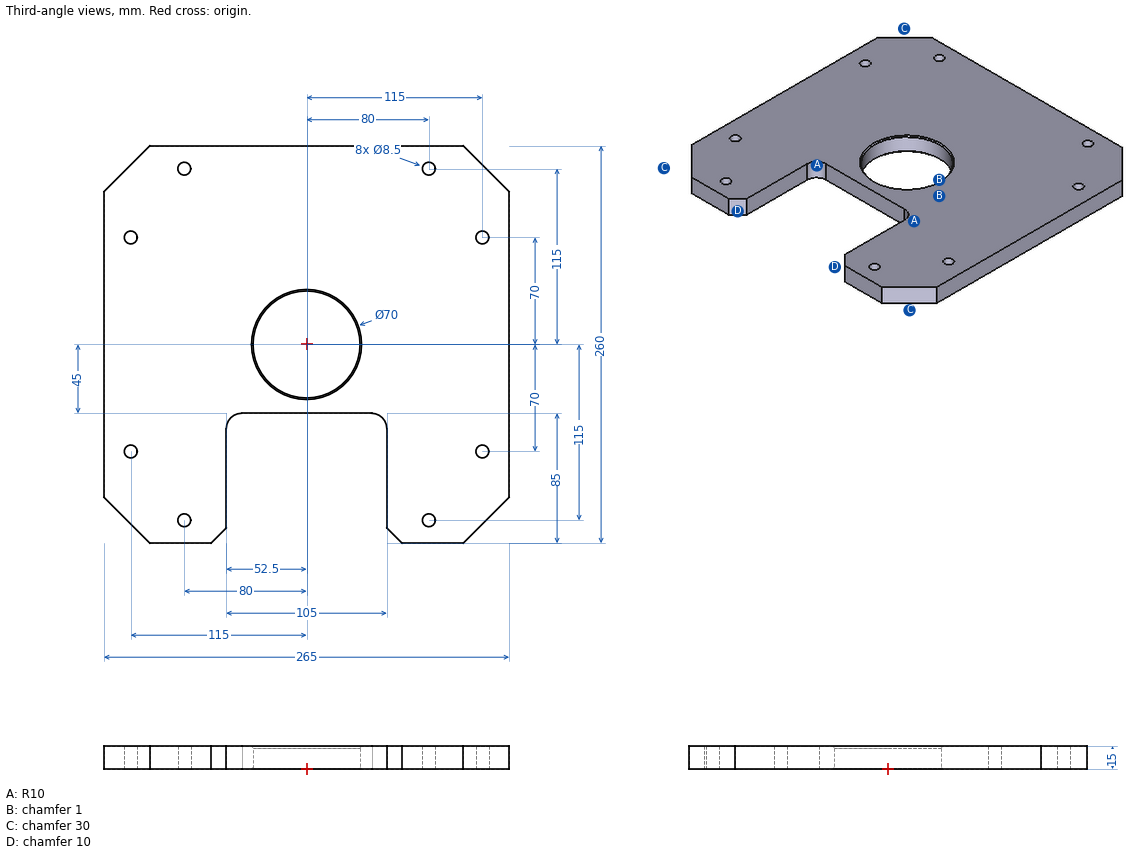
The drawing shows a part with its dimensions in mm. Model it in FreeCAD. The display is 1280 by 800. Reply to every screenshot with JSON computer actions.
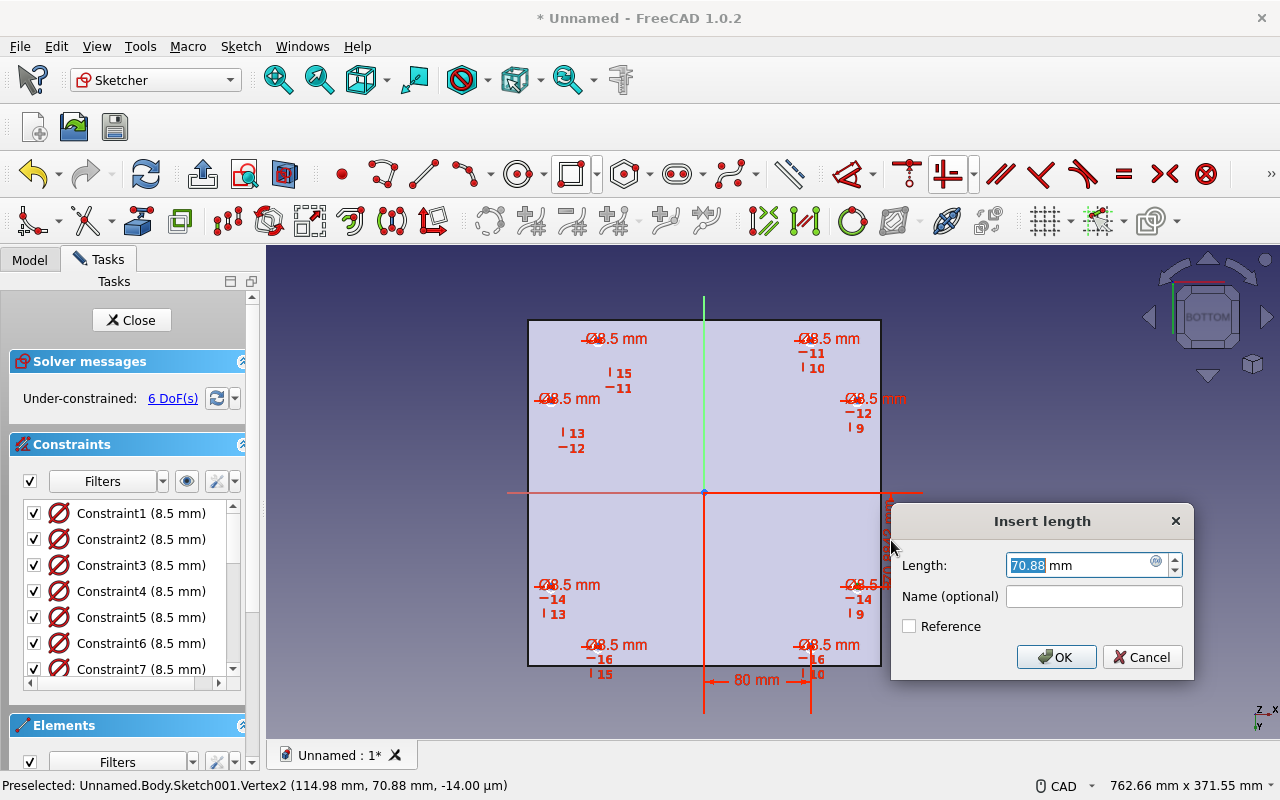
{"action": "type", "text": "70"}
{"action": "key", "text": "Return"}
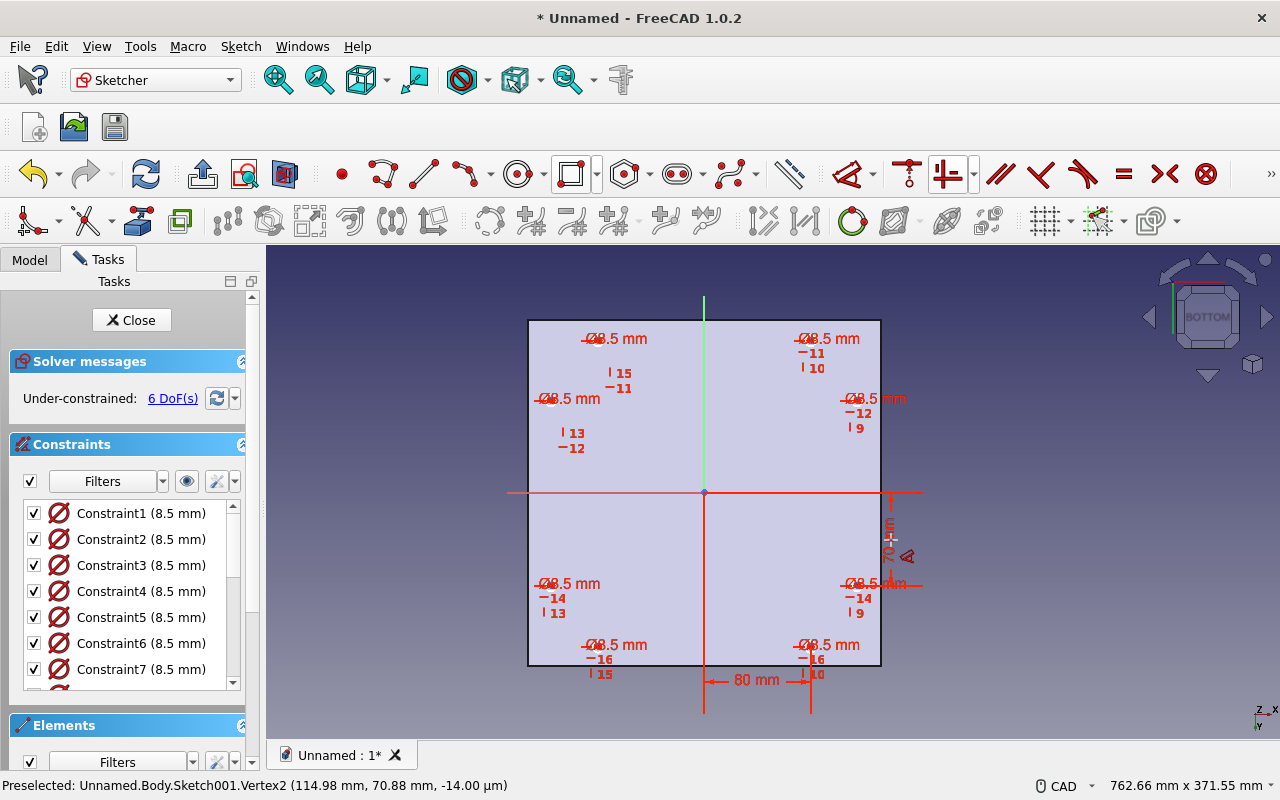
{"action": "left_click", "coordinate": [857, 401]}
{"action": "left_click", "coordinate": [891, 447]}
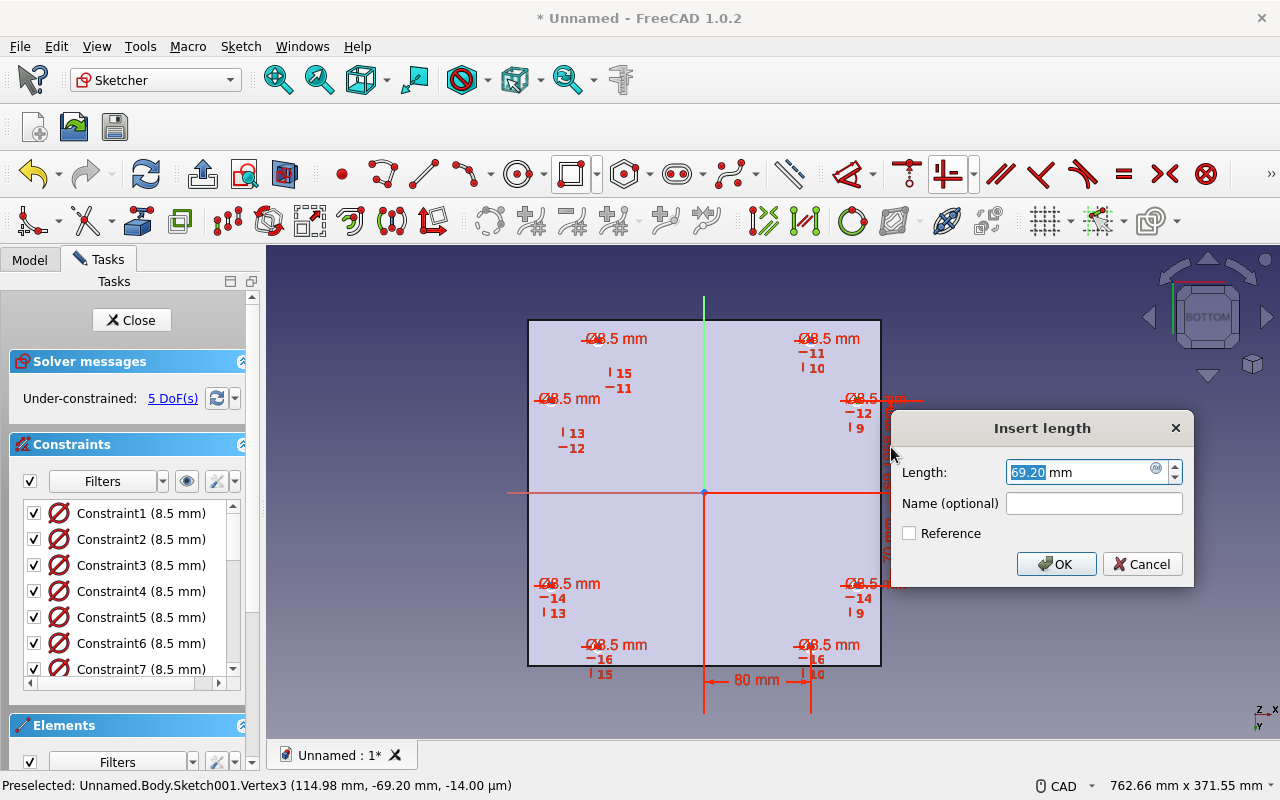
{"action": "type", "text": "70"}
{"action": "key", "text": "Return"}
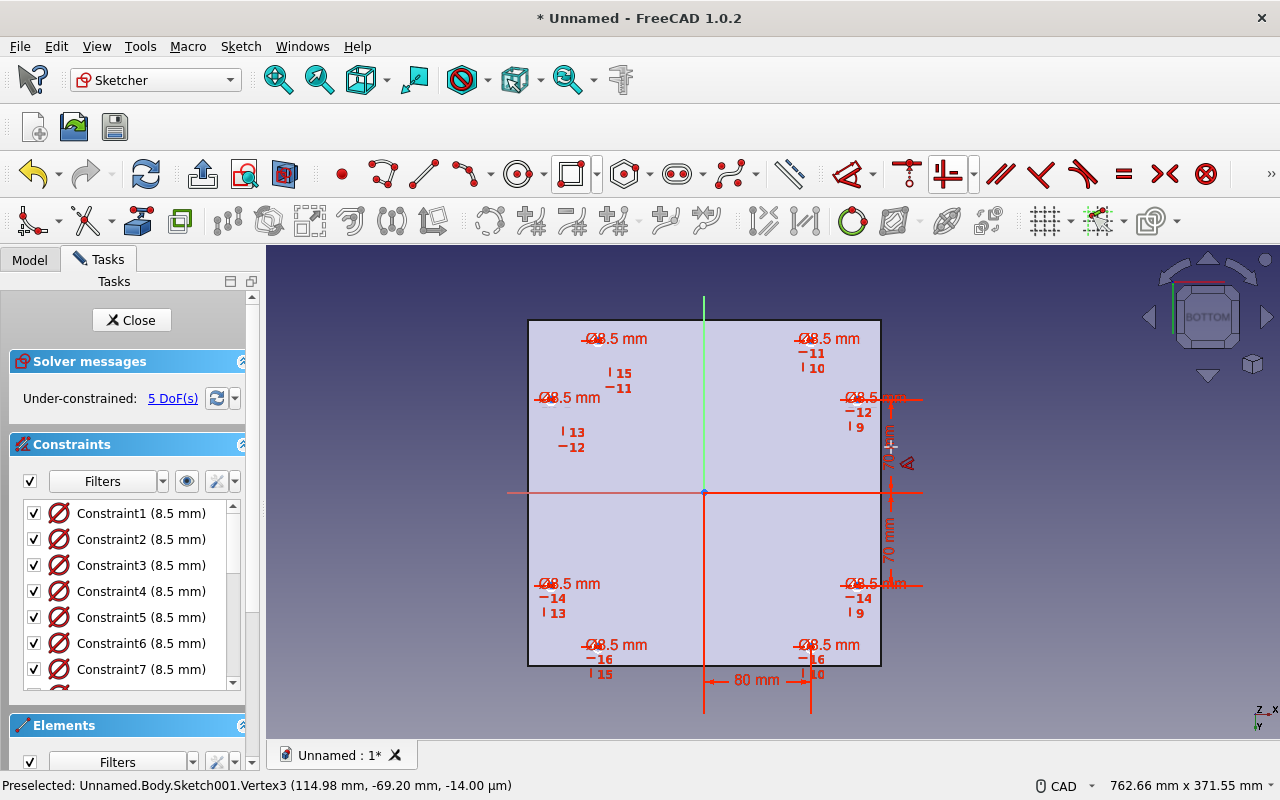
{"action": "left_click", "coordinate": [598, 341]}
{"action": "left_click", "coordinate": [651, 307]}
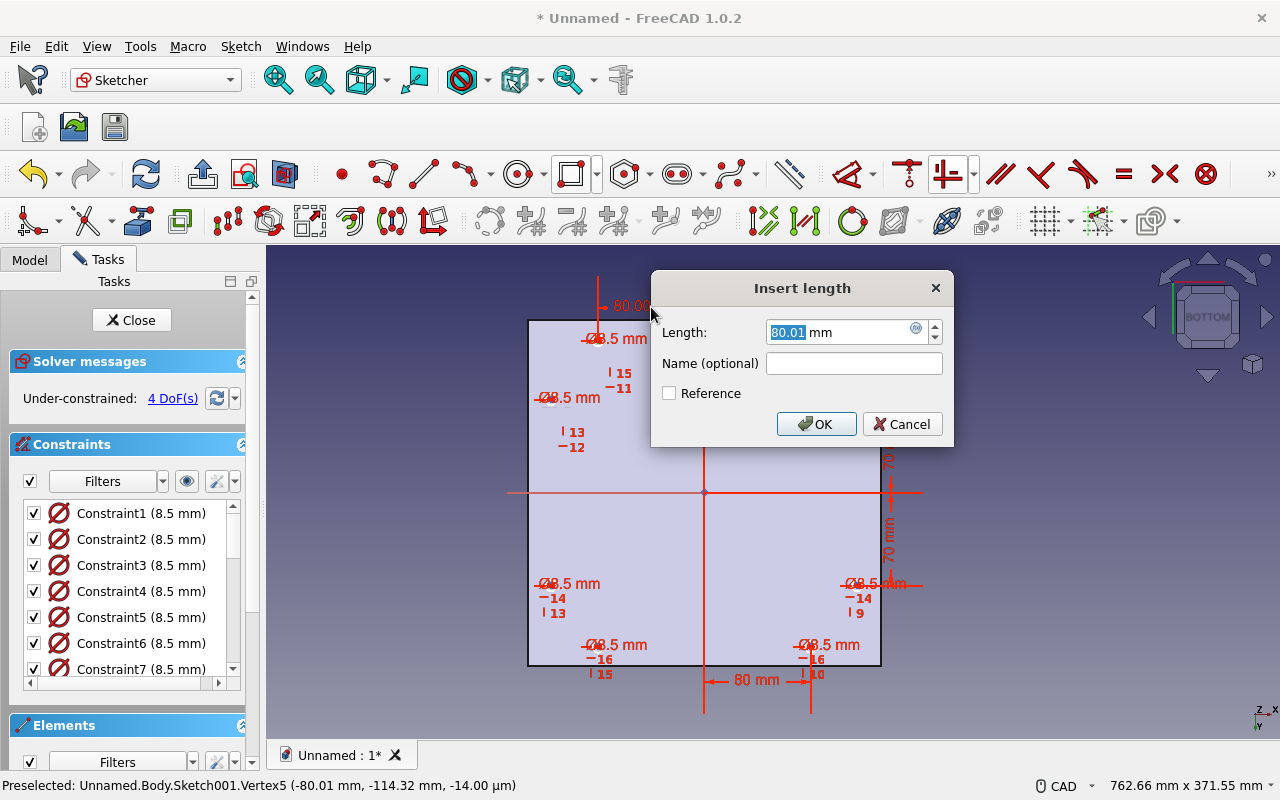
{"action": "type", "text": "80"}
{"action": "key", "text": "Return"}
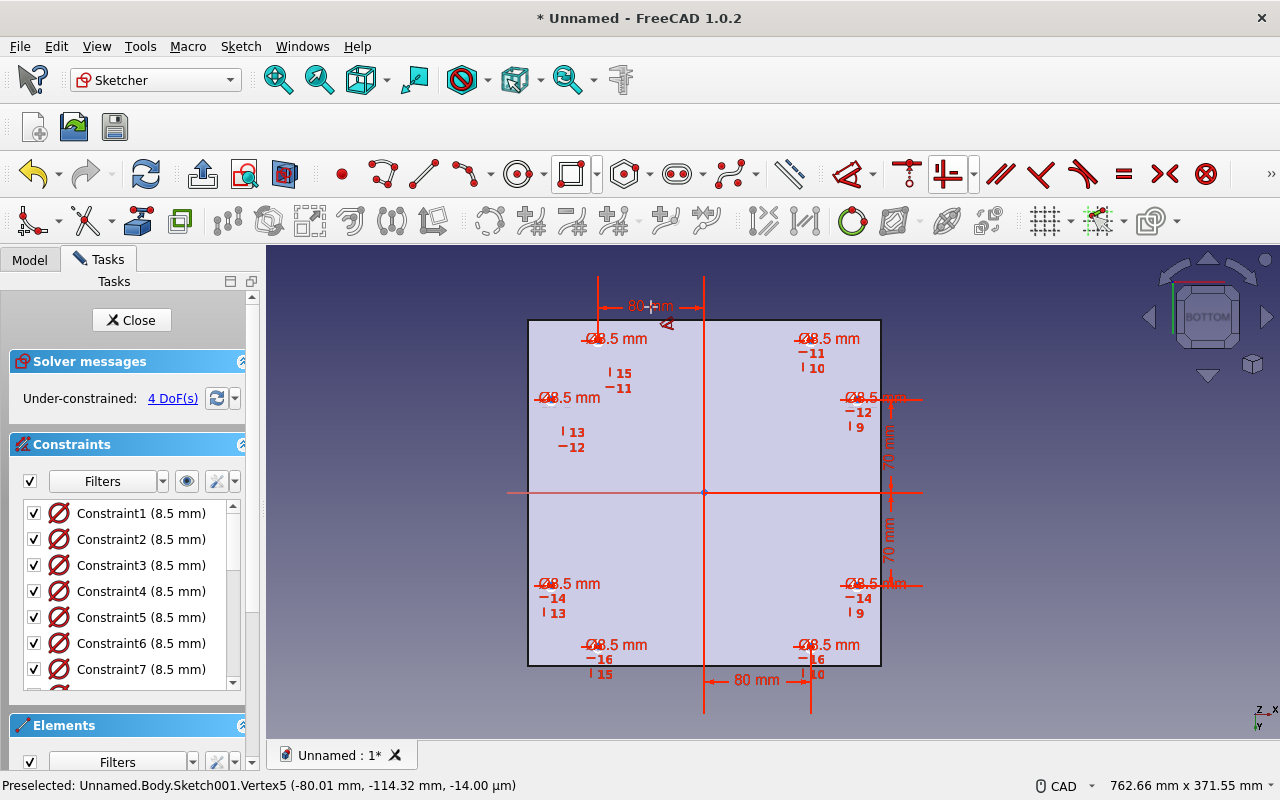
{"action": "left_click", "coordinate": [811, 647]}
{"action": "left_click", "coordinate": [845, 570]}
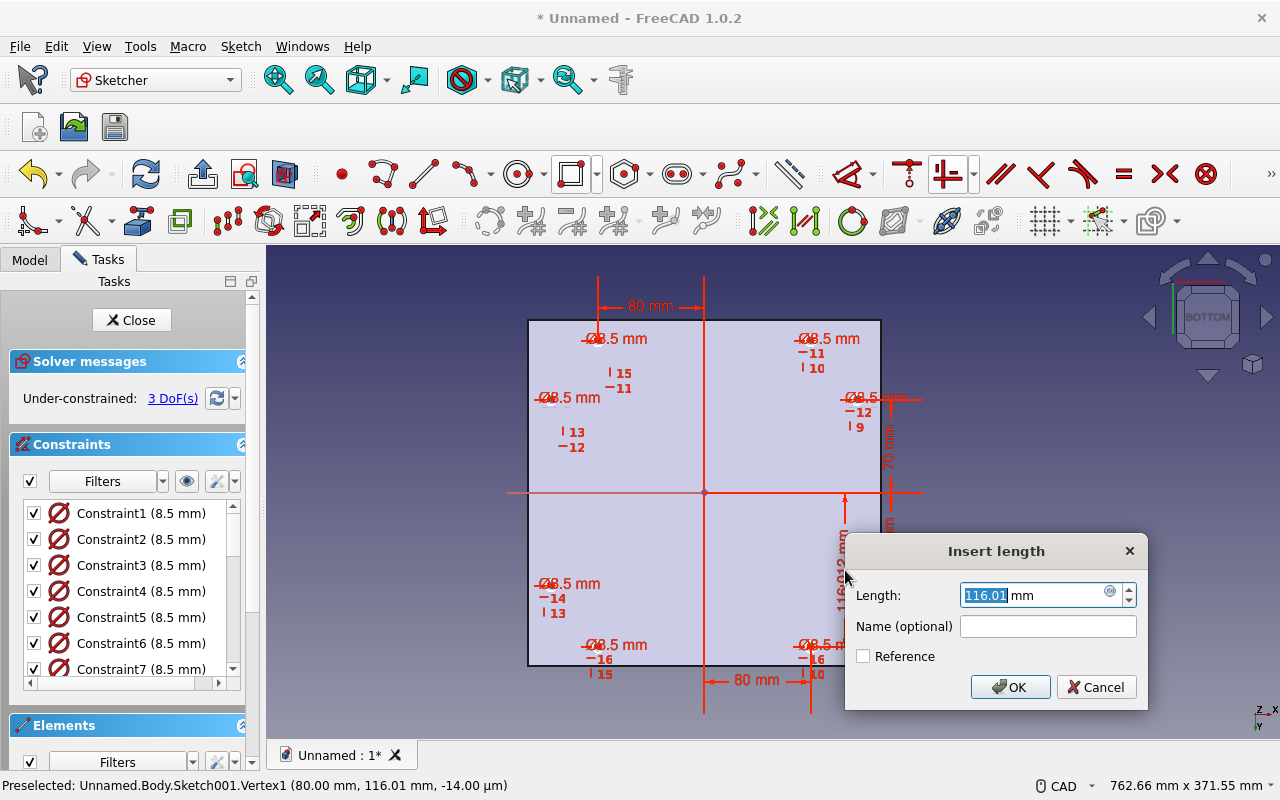
{"action": "type", "text": "115"}
{"action": "key", "text": "Return"}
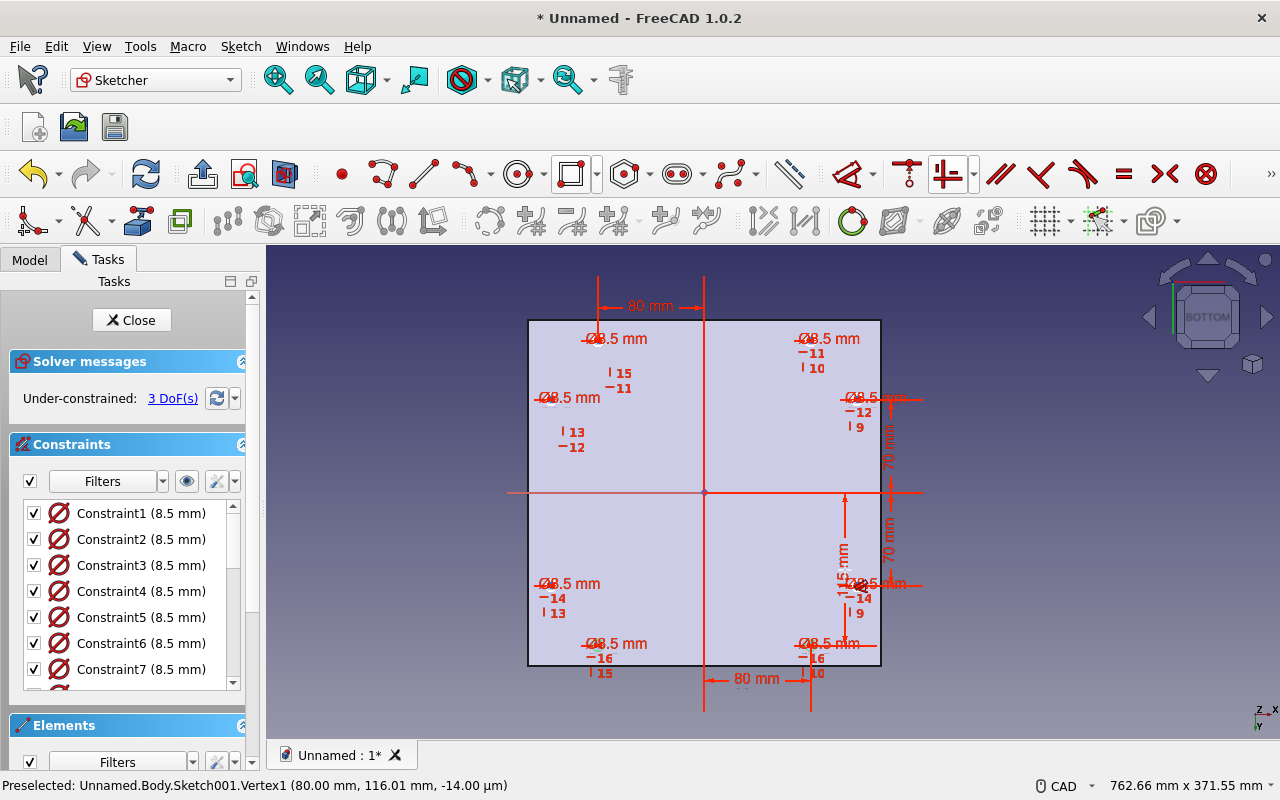
{"action": "left_click", "coordinate": [857, 586]}
{"action": "left_click", "coordinate": [781, 620]}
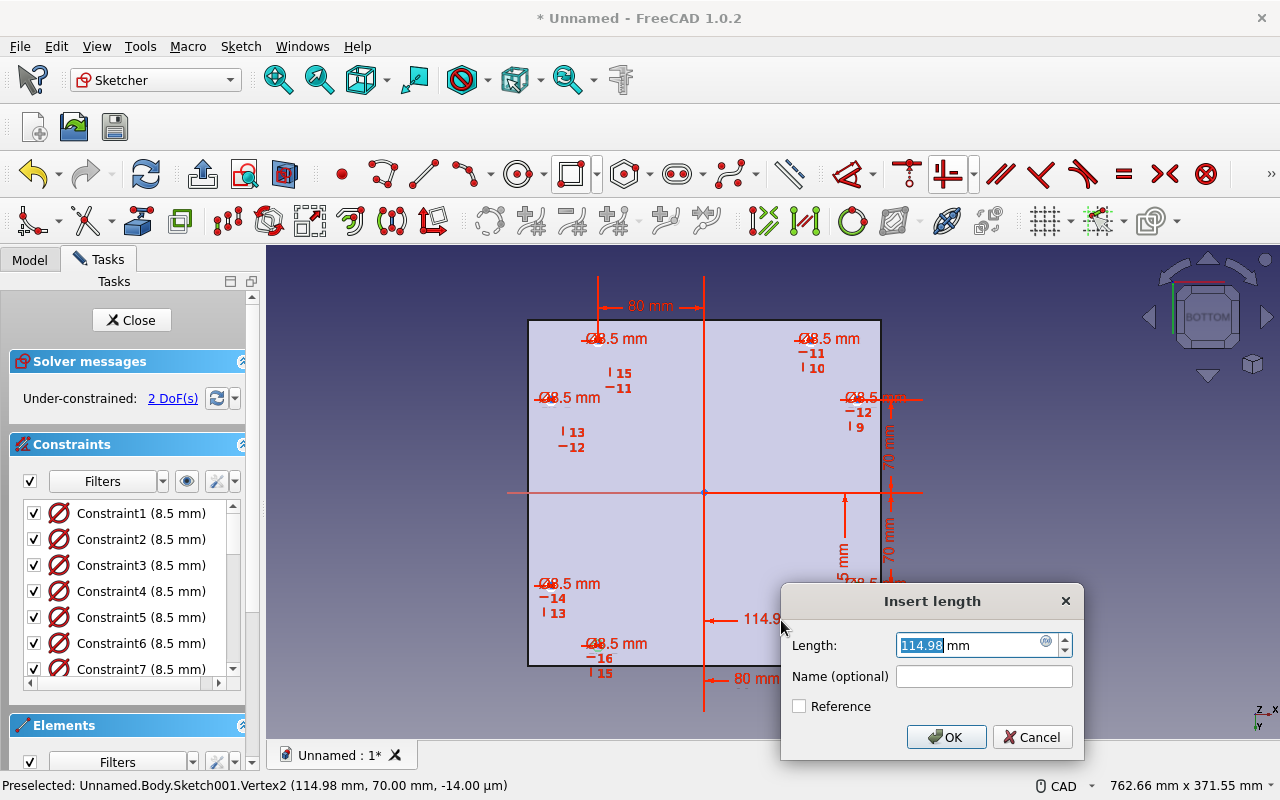
{"action": "type", "text": "115"}
{"action": "key", "text": "Return"}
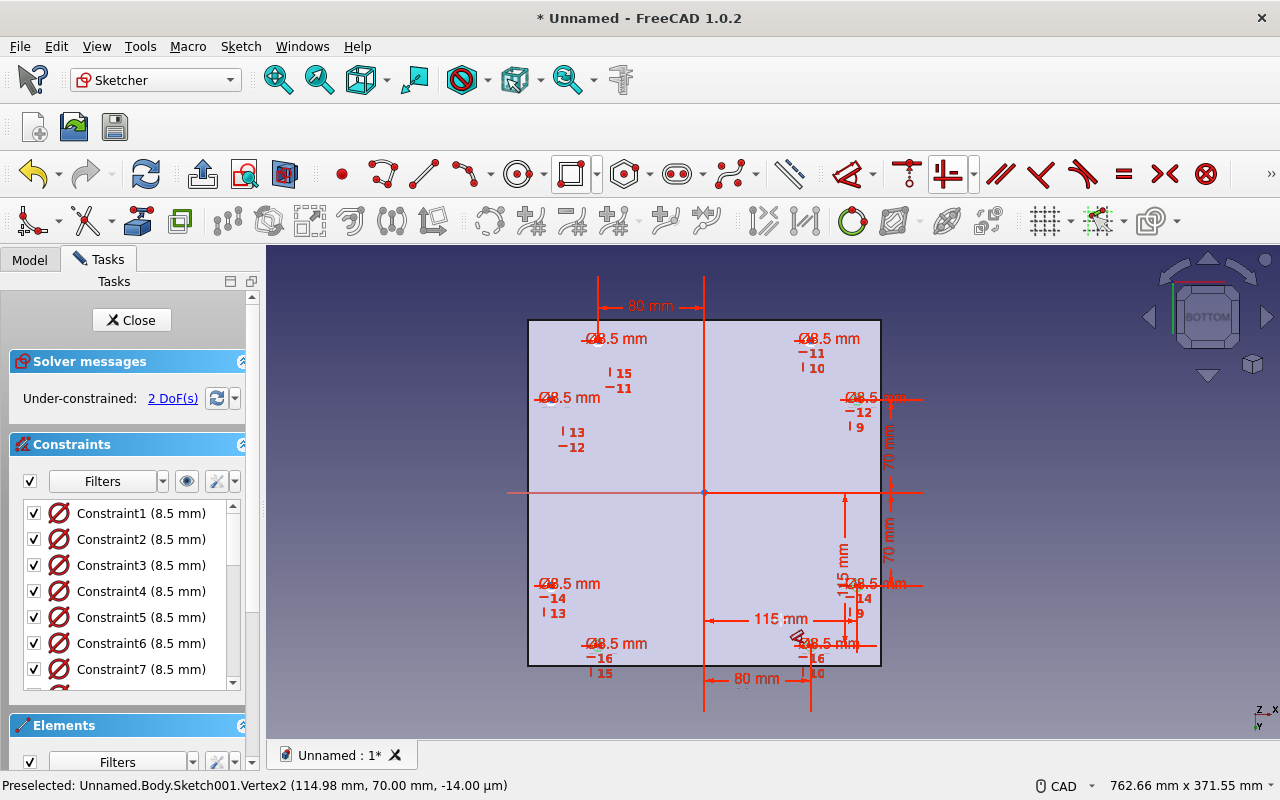
{"action": "left_click", "coordinate": [811, 341]}
{"action": "left_click", "coordinate": [845, 417]}